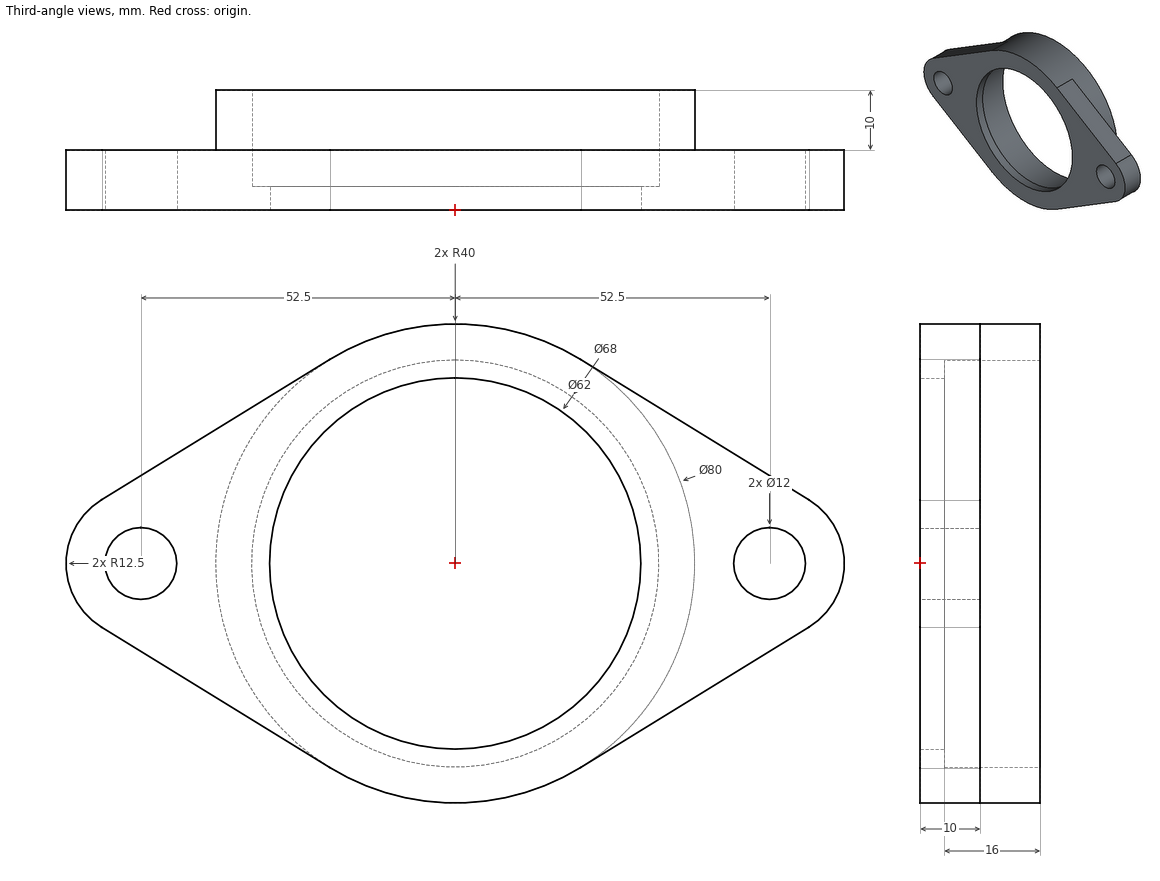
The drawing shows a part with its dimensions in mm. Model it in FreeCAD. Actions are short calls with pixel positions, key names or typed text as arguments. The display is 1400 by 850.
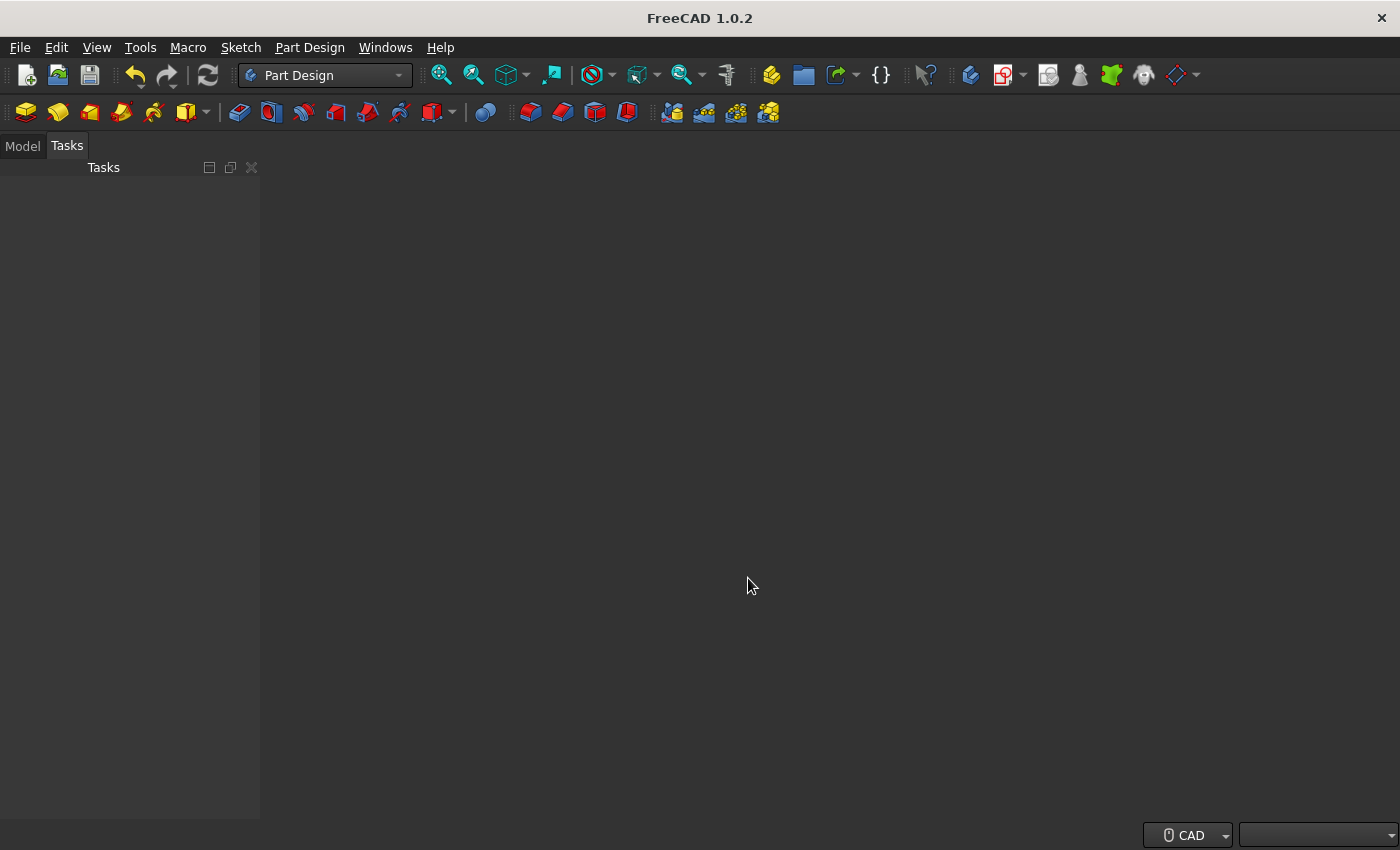
click(26, 76)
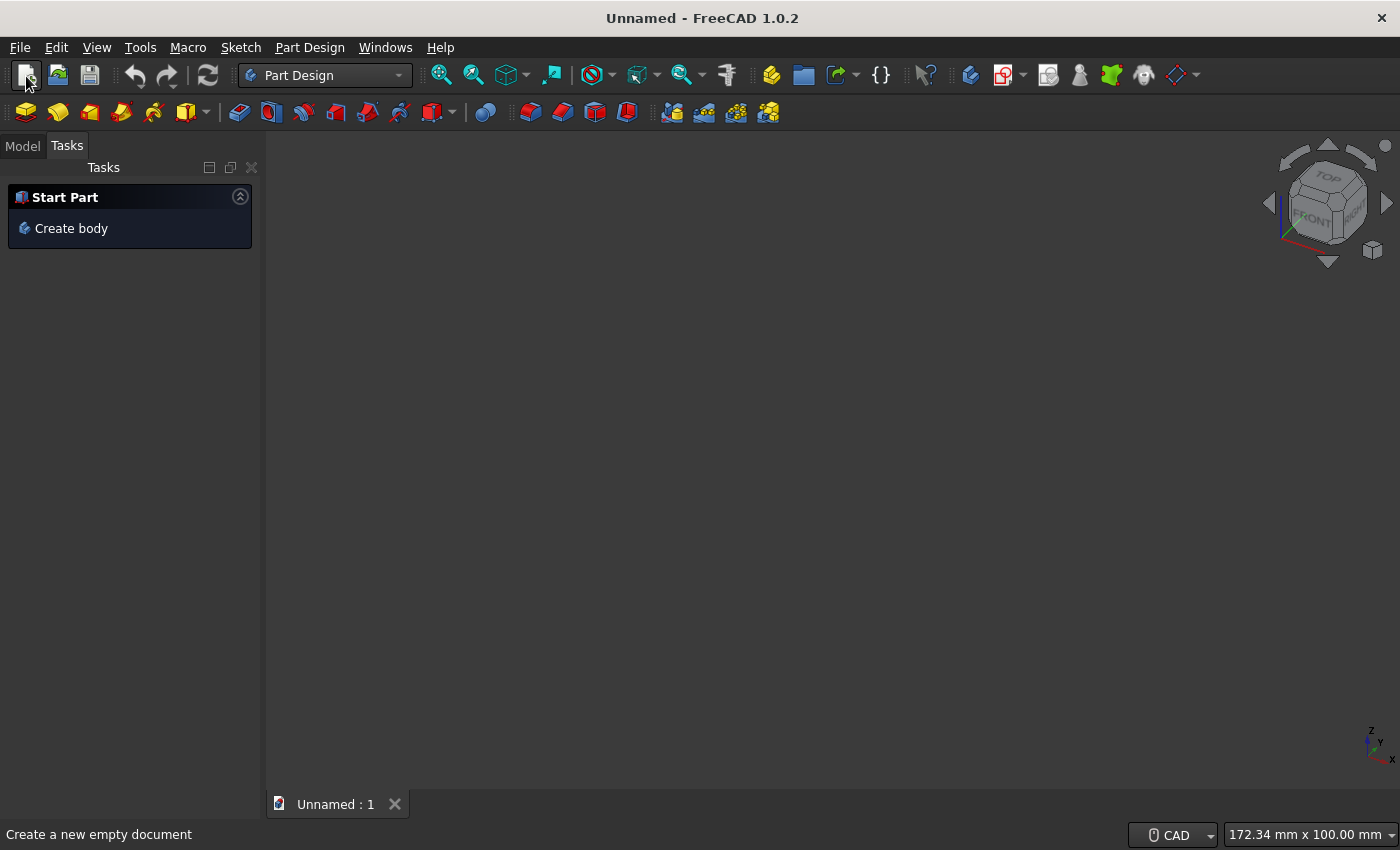
click(1004, 76)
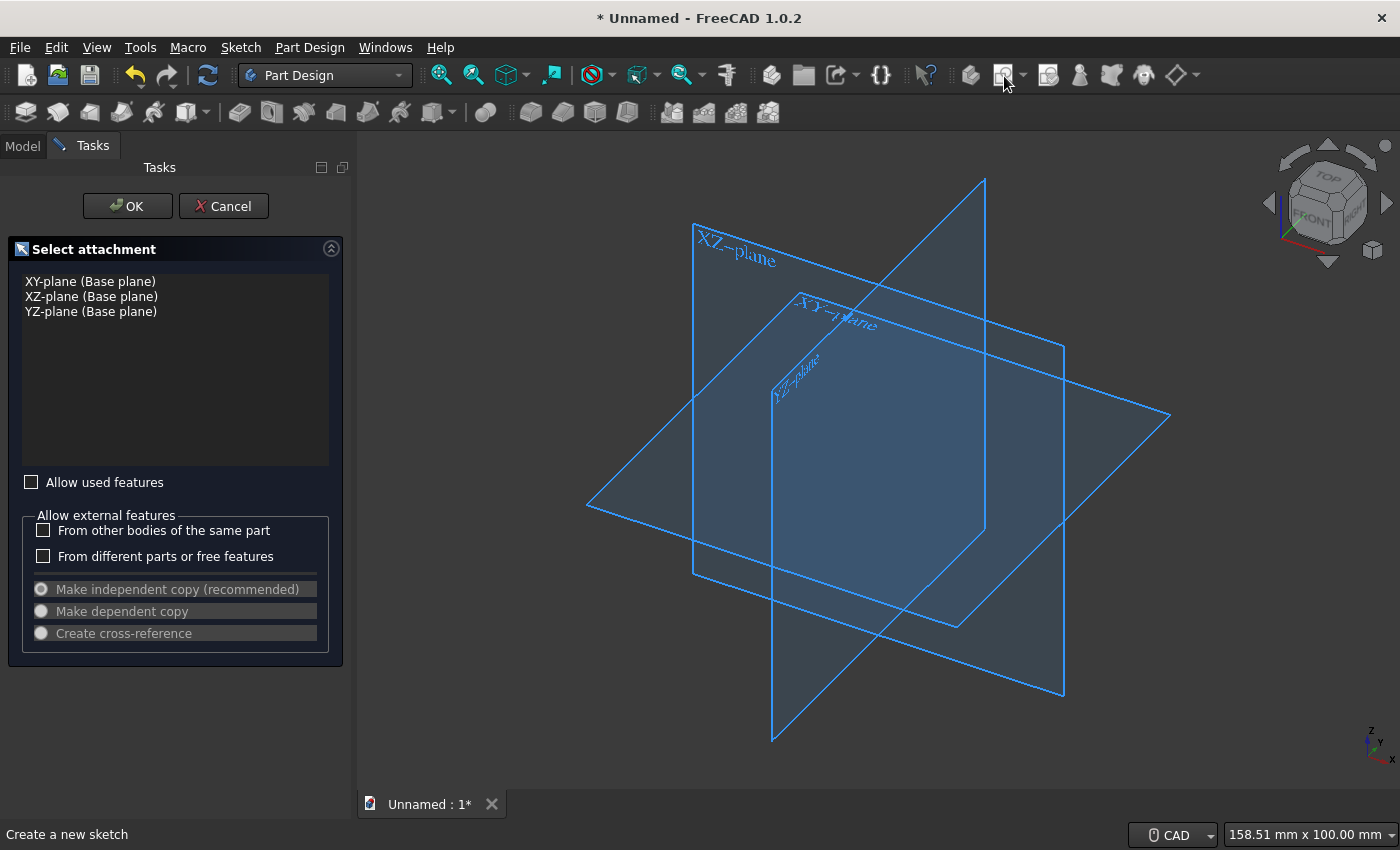
click(82, 296)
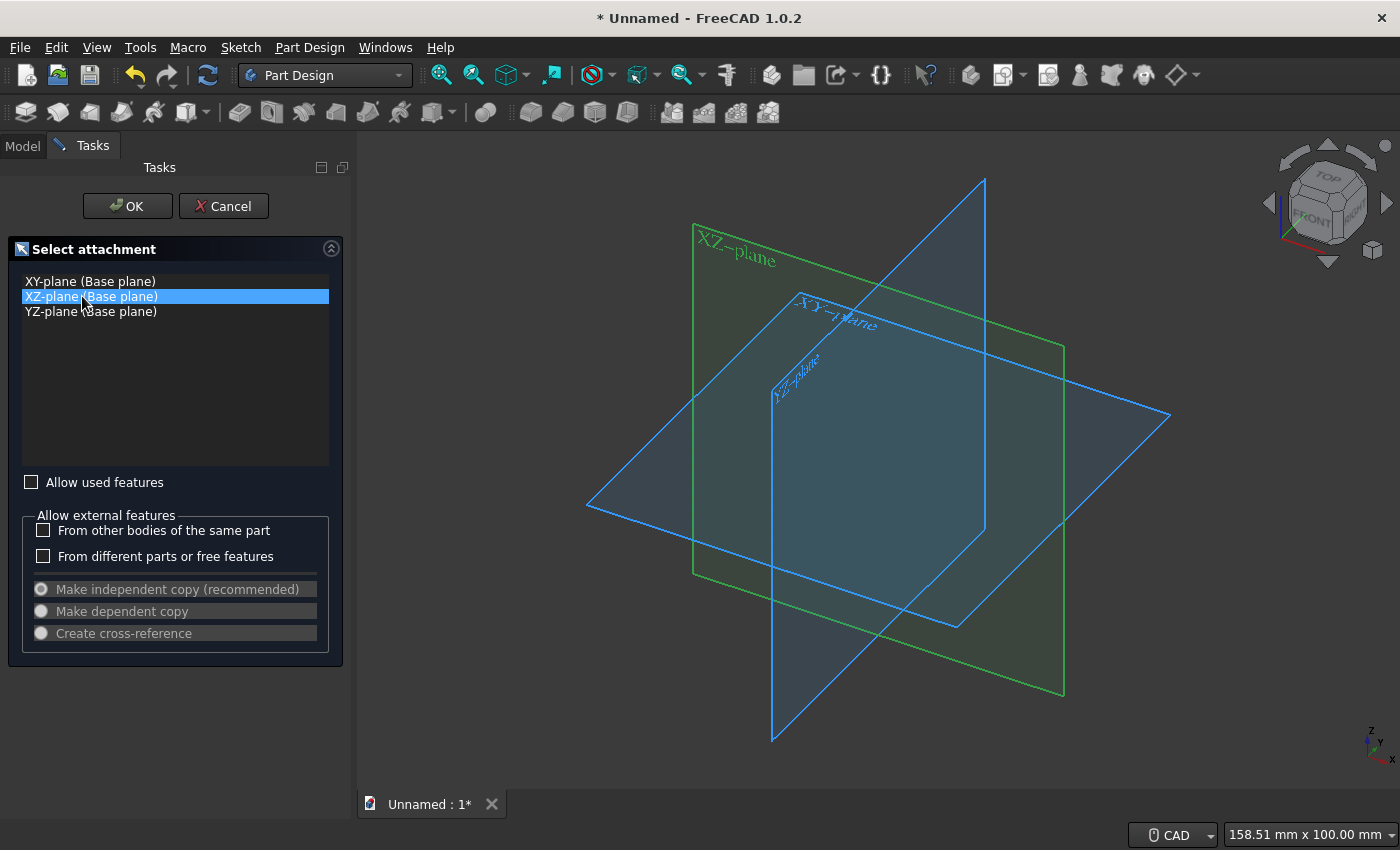
click(128, 206)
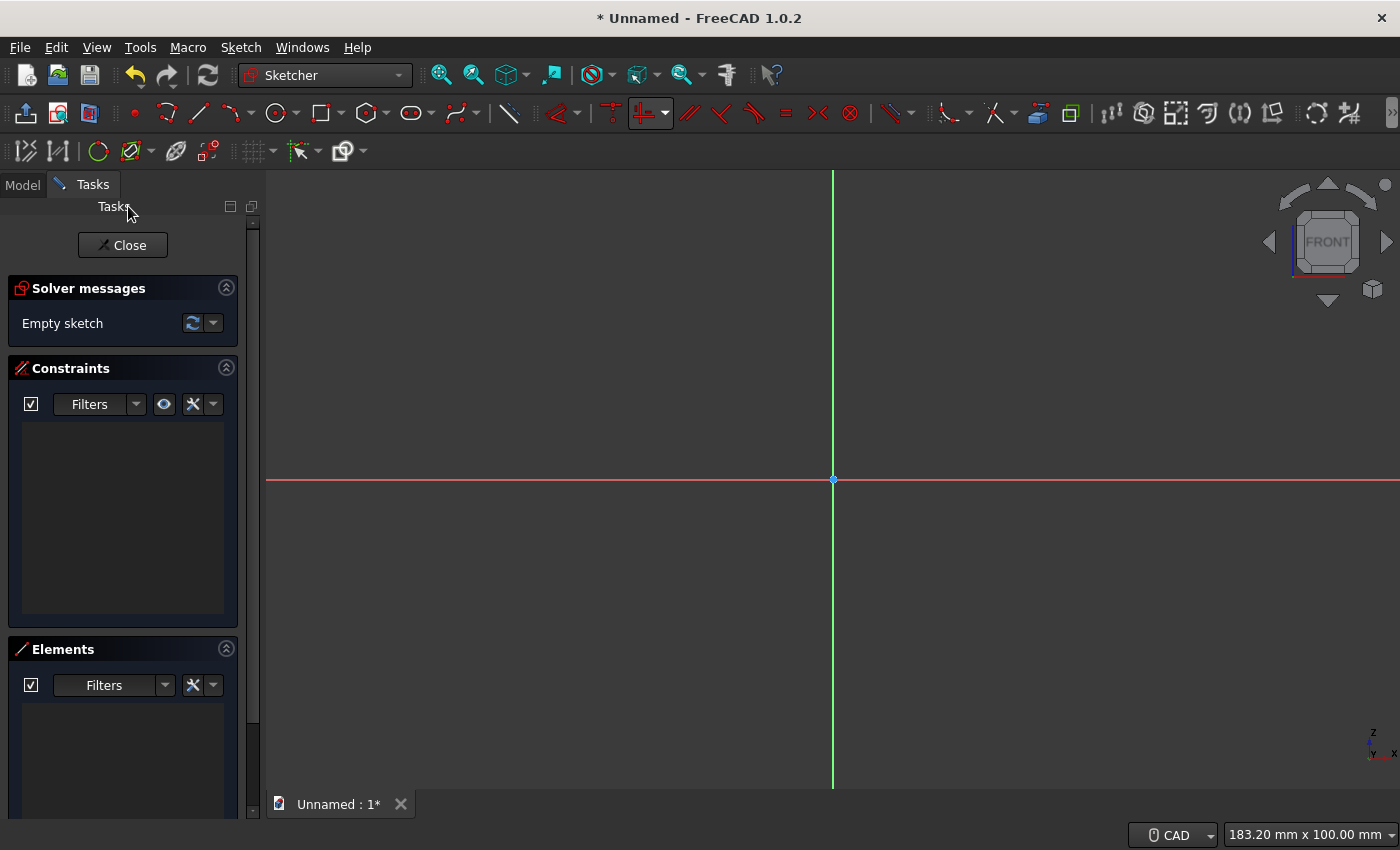
scroll(455, 480, down, 1)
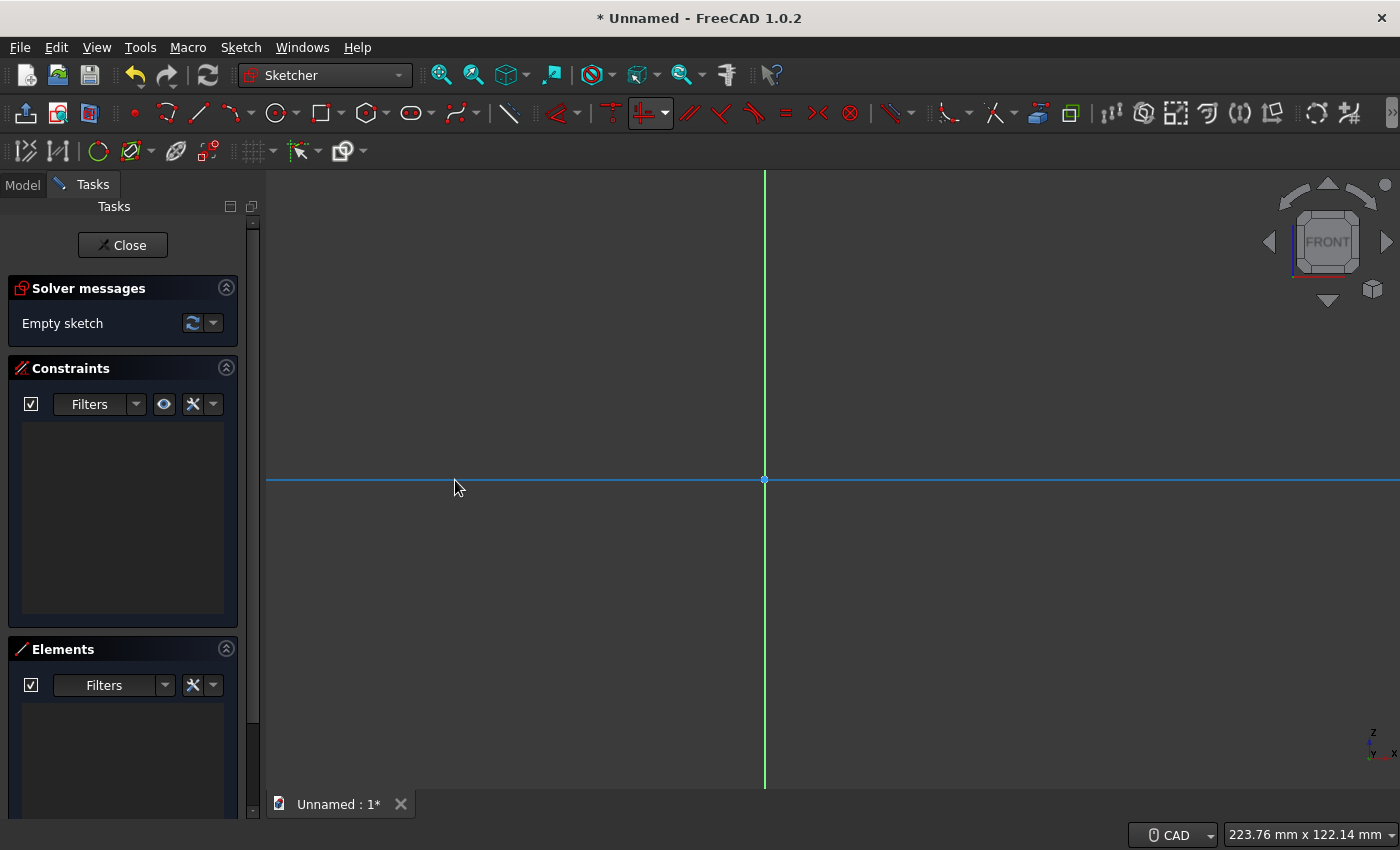
click(200, 114)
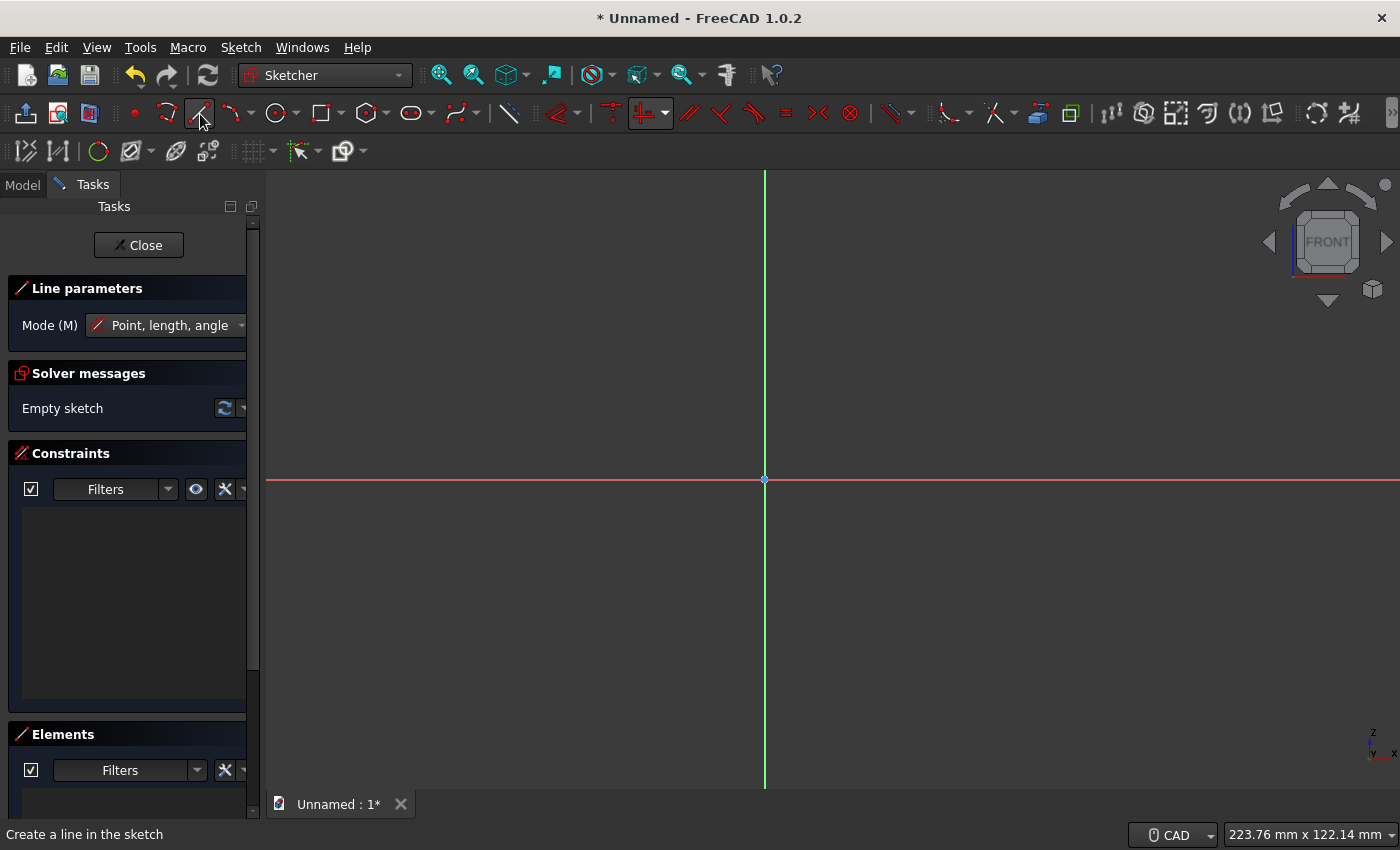
click(658, 652)
click(465, 534)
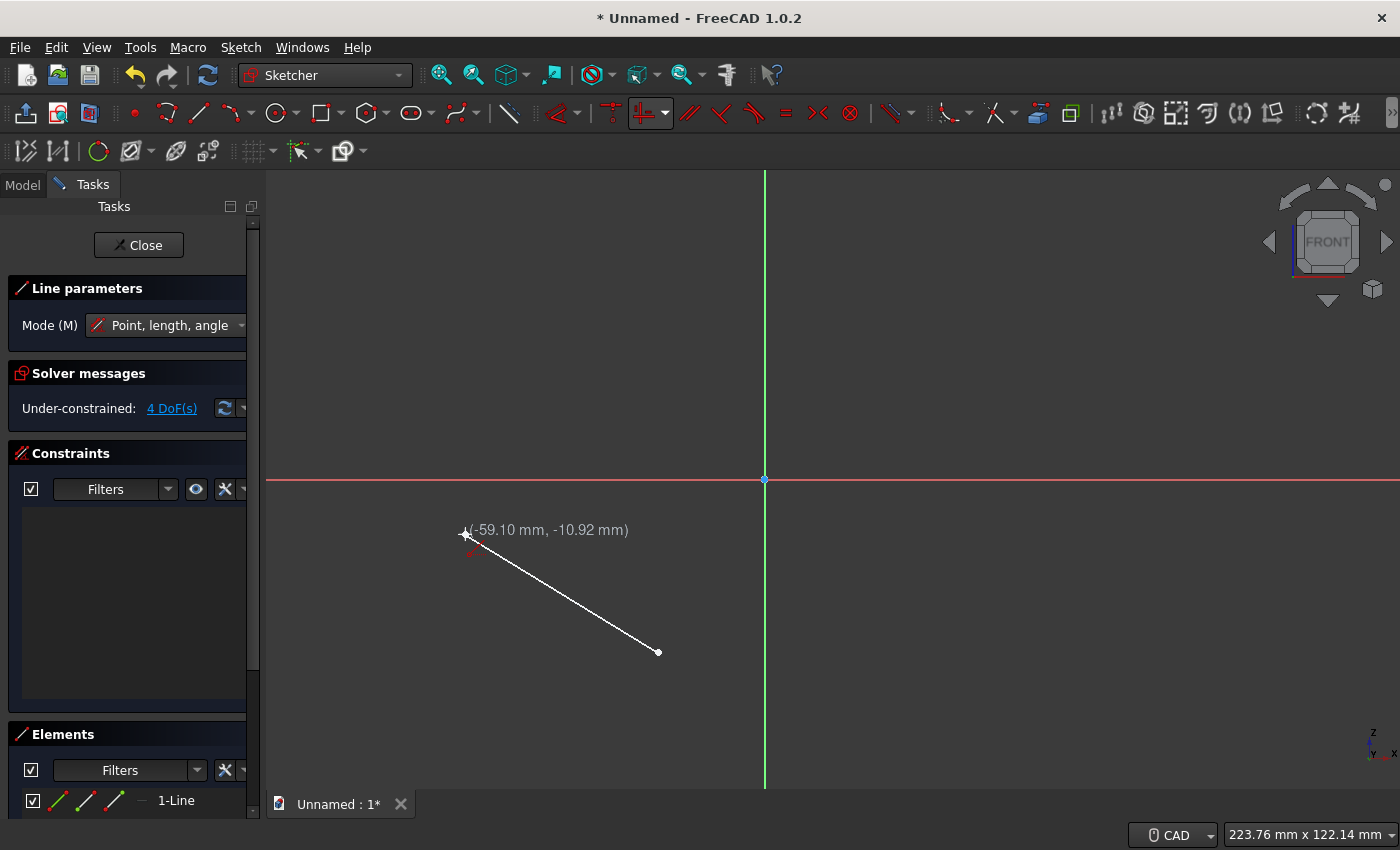
click(465, 426)
click(658, 307)